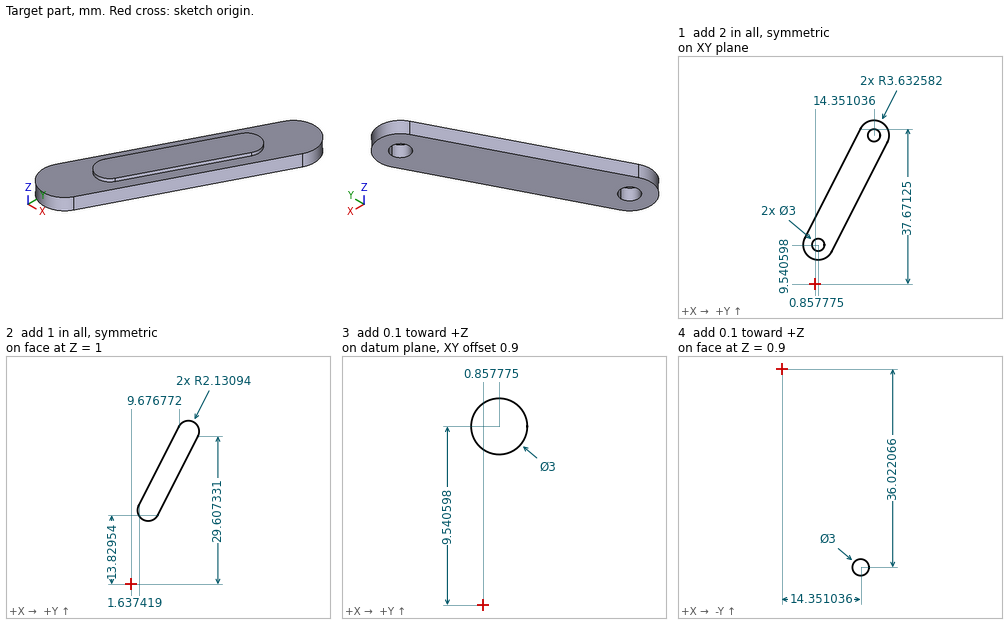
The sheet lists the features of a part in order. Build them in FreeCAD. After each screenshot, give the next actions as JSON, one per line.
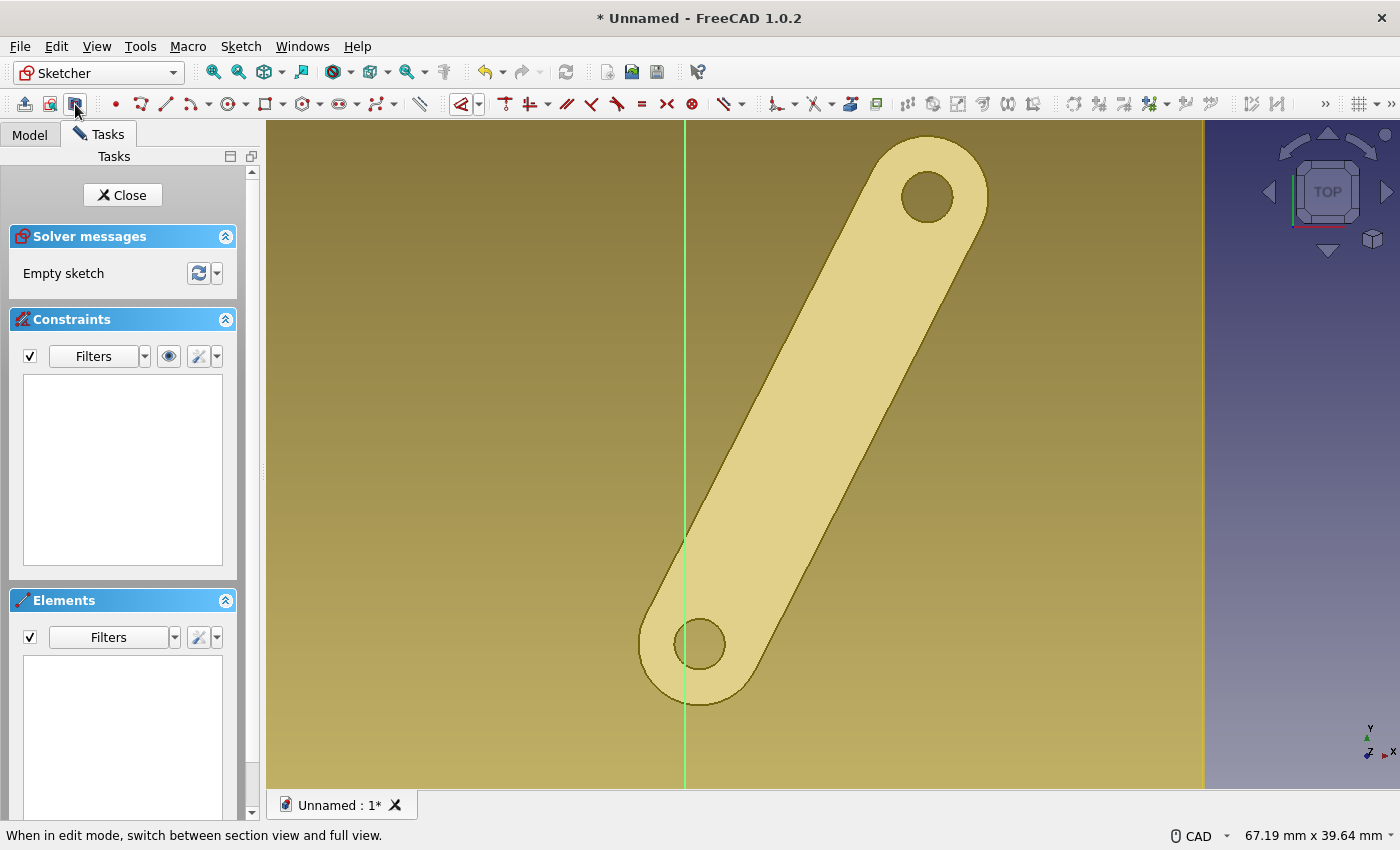
{"action": "scroll", "coordinate": [692, 668], "scroll_direction": "up", "scroll_amount": 11}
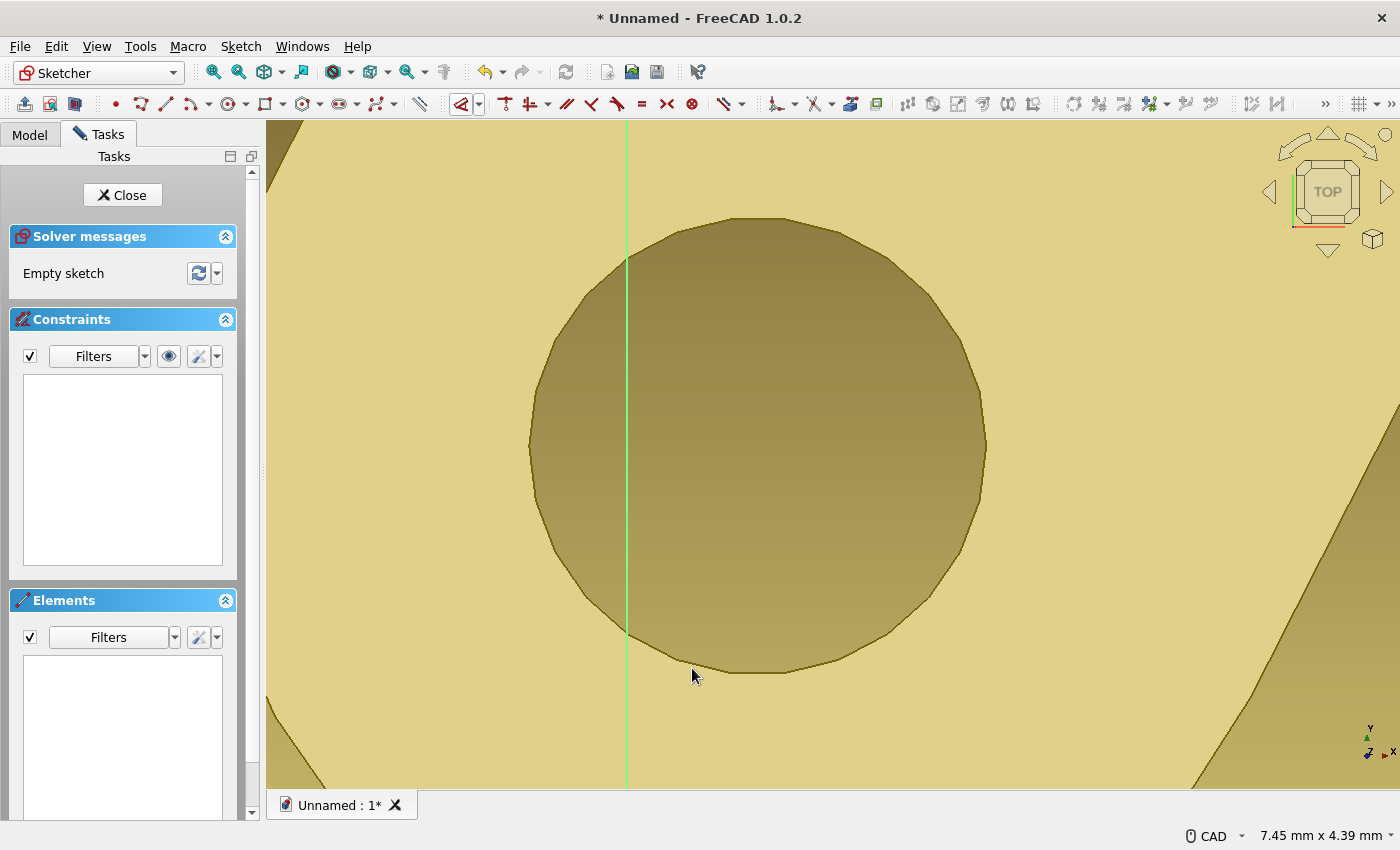
{"action": "key", "text": "g c"}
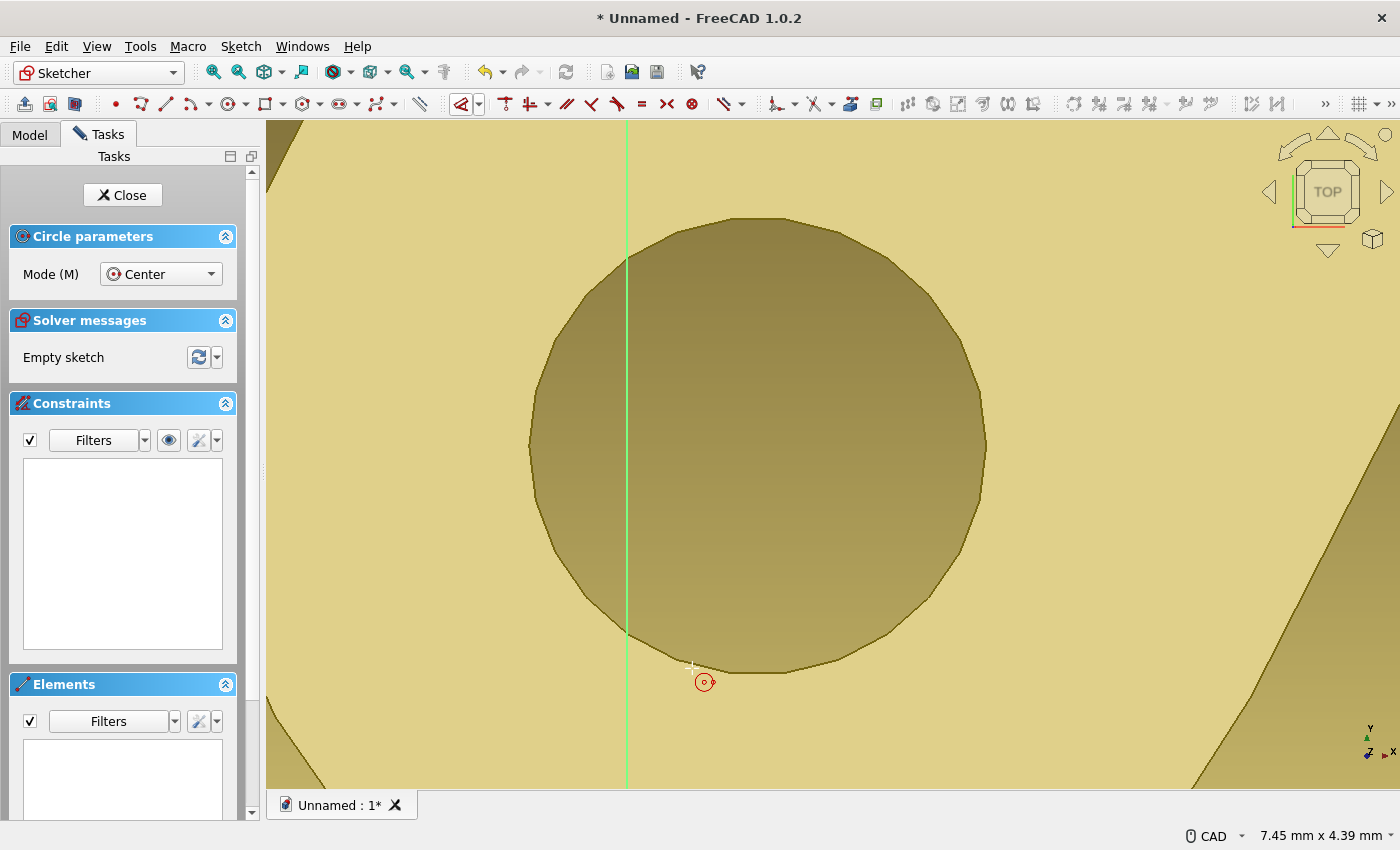
{"action": "left_click", "coordinate": [758, 446]}
{"action": "left_click", "coordinate": [919, 285]}
{"action": "key", "text": "Escape"}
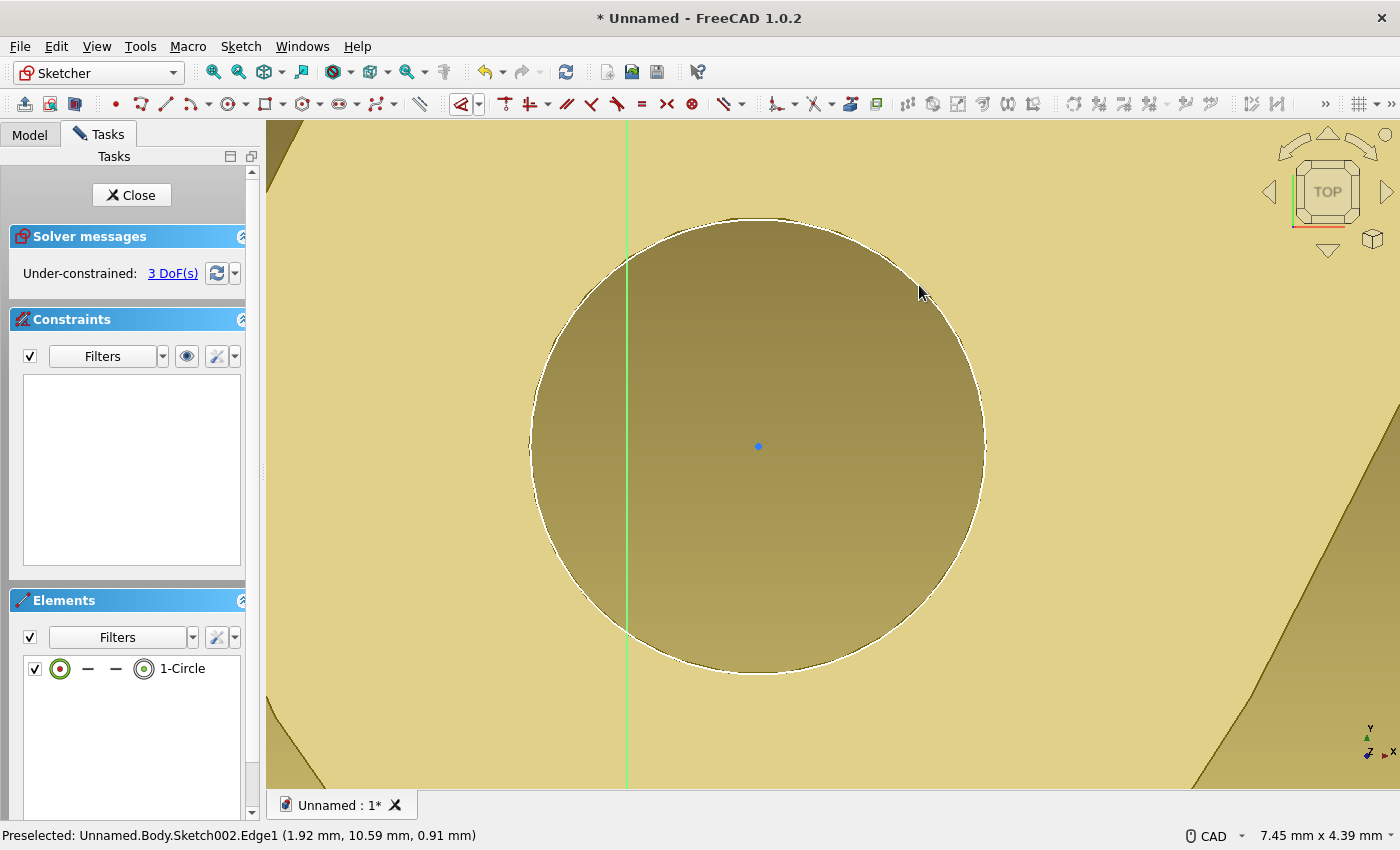
{"action": "left_click", "coordinate": [919, 286]}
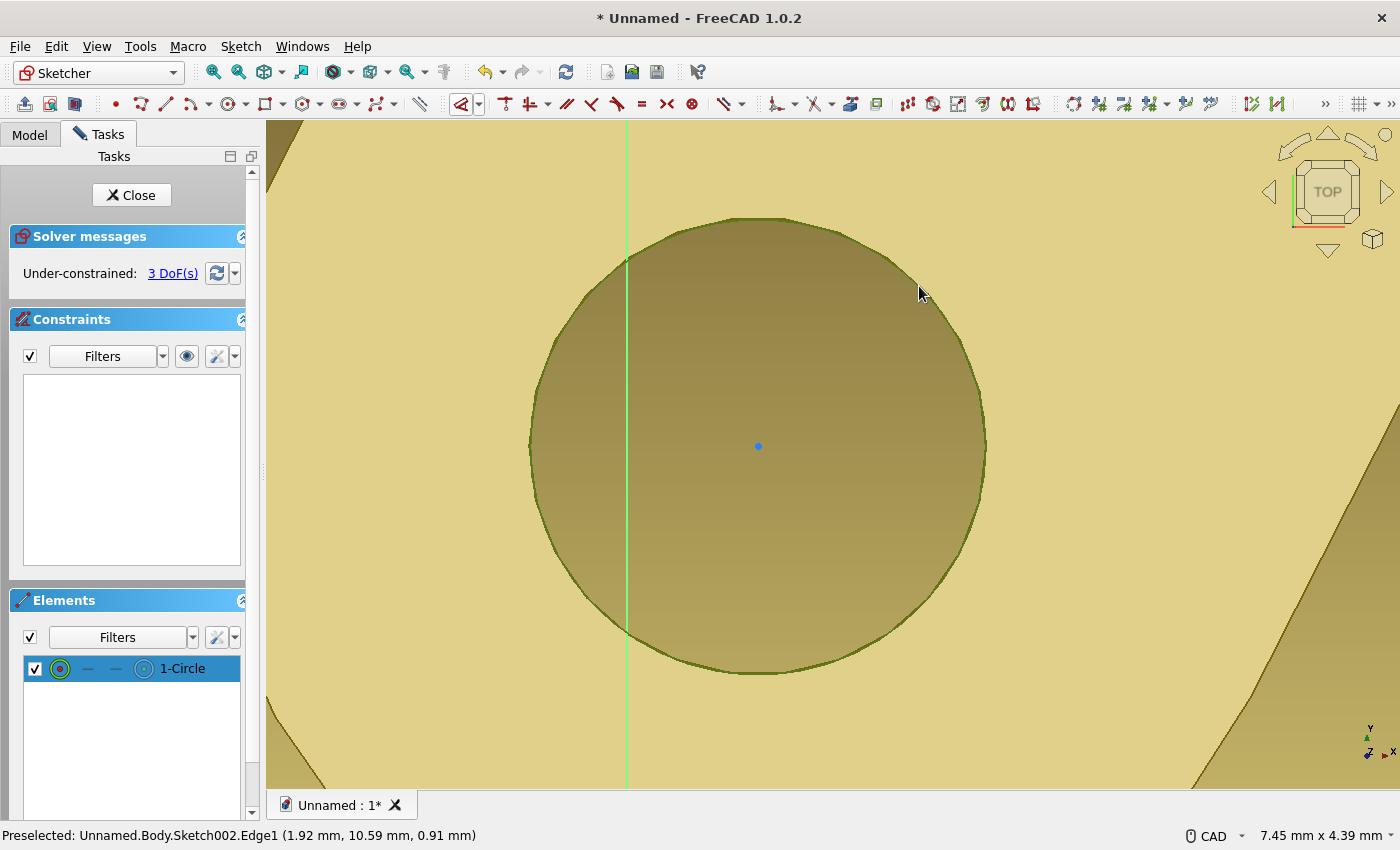
{"action": "key", "text": "k o"}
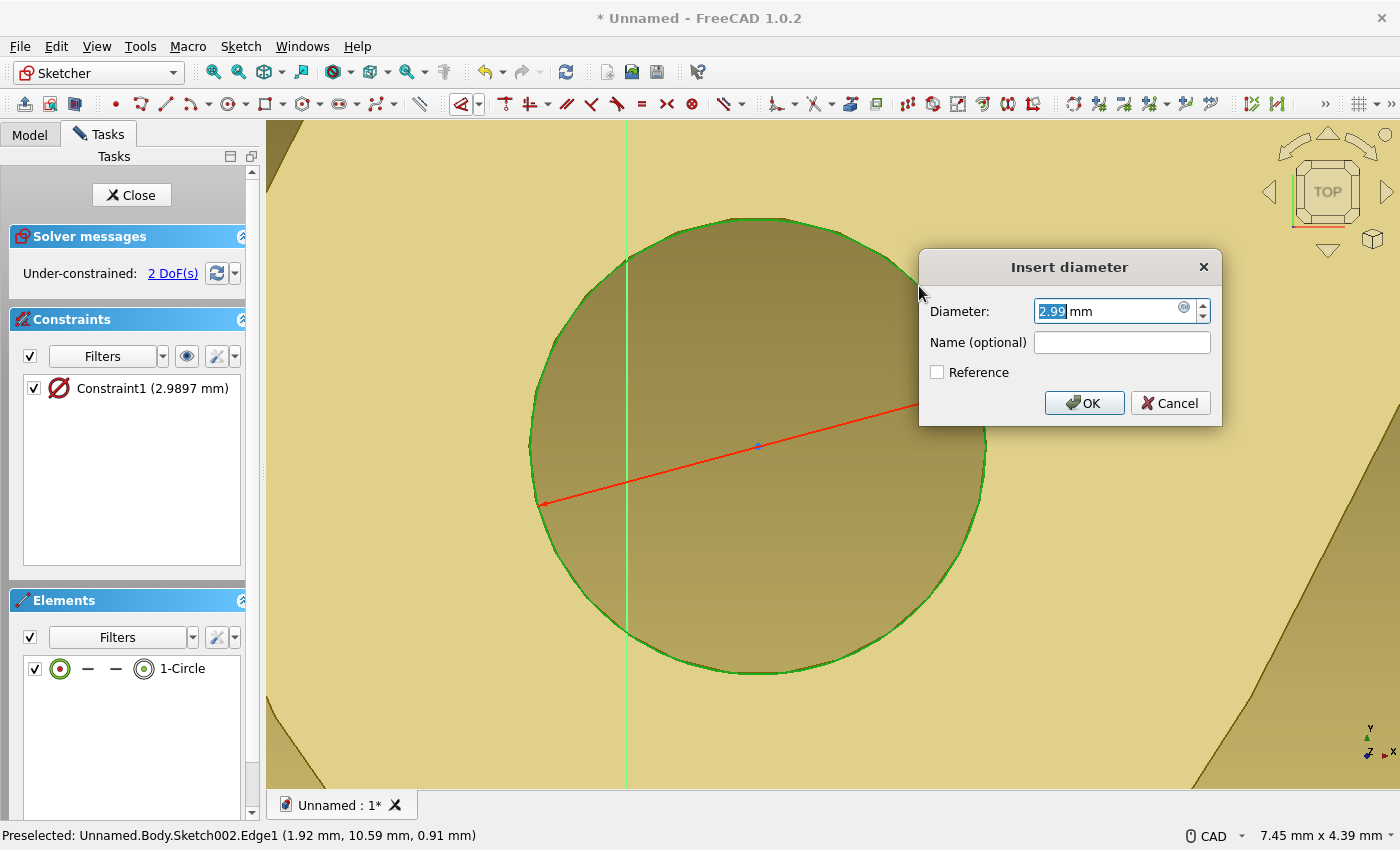
{"action": "type", "text": "3"}
{"action": "key", "text": "Return"}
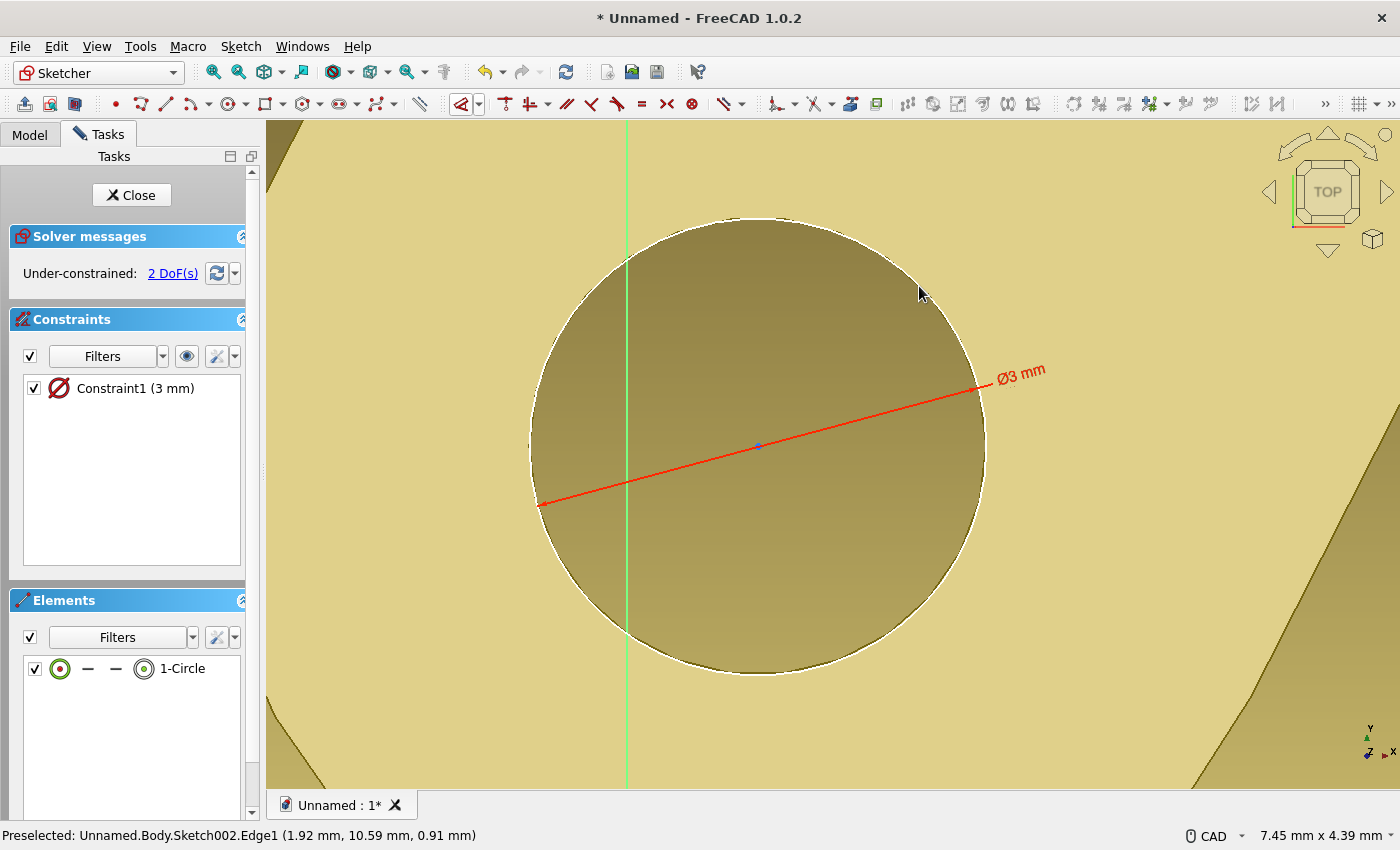
{"action": "left_click", "coordinate": [758, 447]}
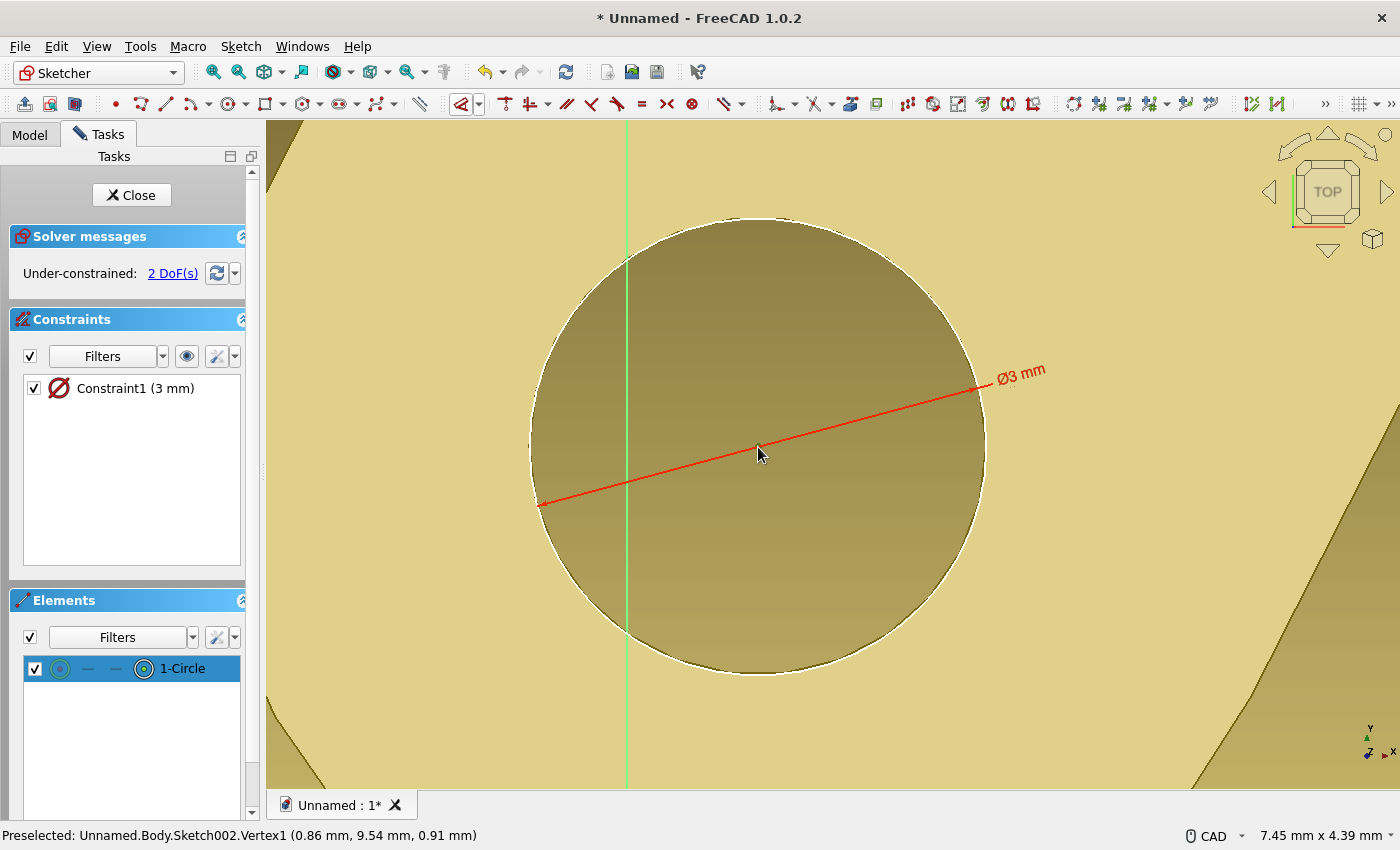
{"action": "key", "text": "l"}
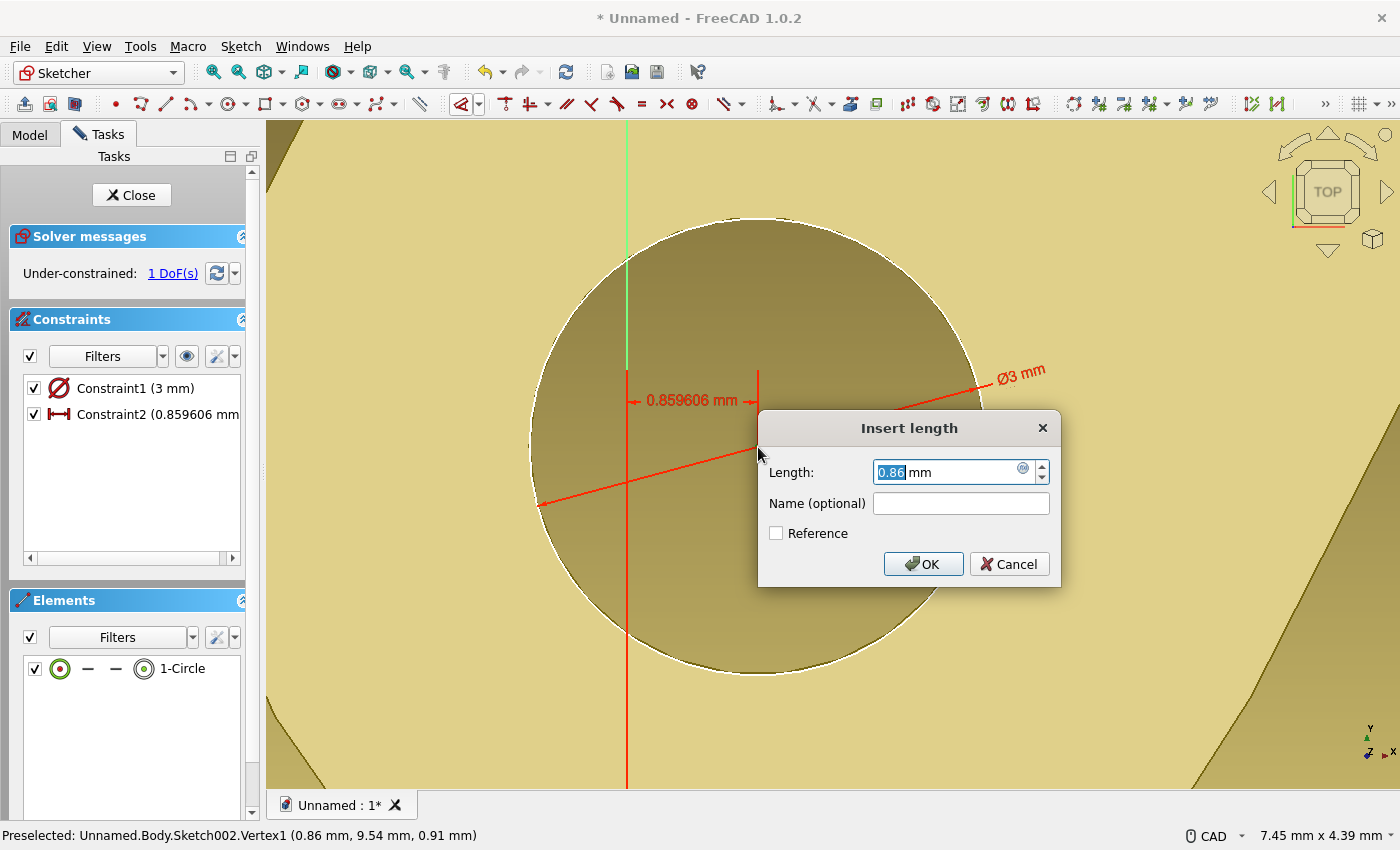
{"action": "type", "text": "0.857775"}
{"action": "key", "text": "Return"}